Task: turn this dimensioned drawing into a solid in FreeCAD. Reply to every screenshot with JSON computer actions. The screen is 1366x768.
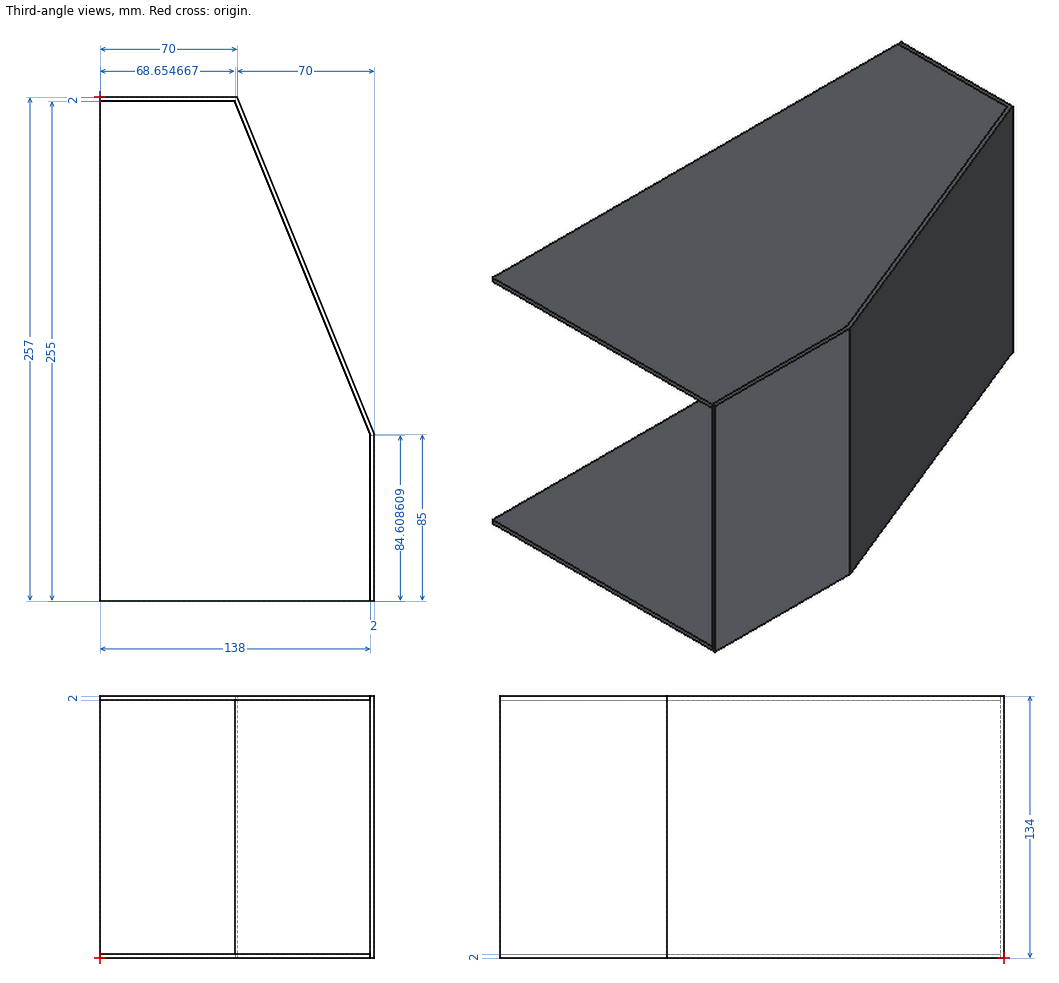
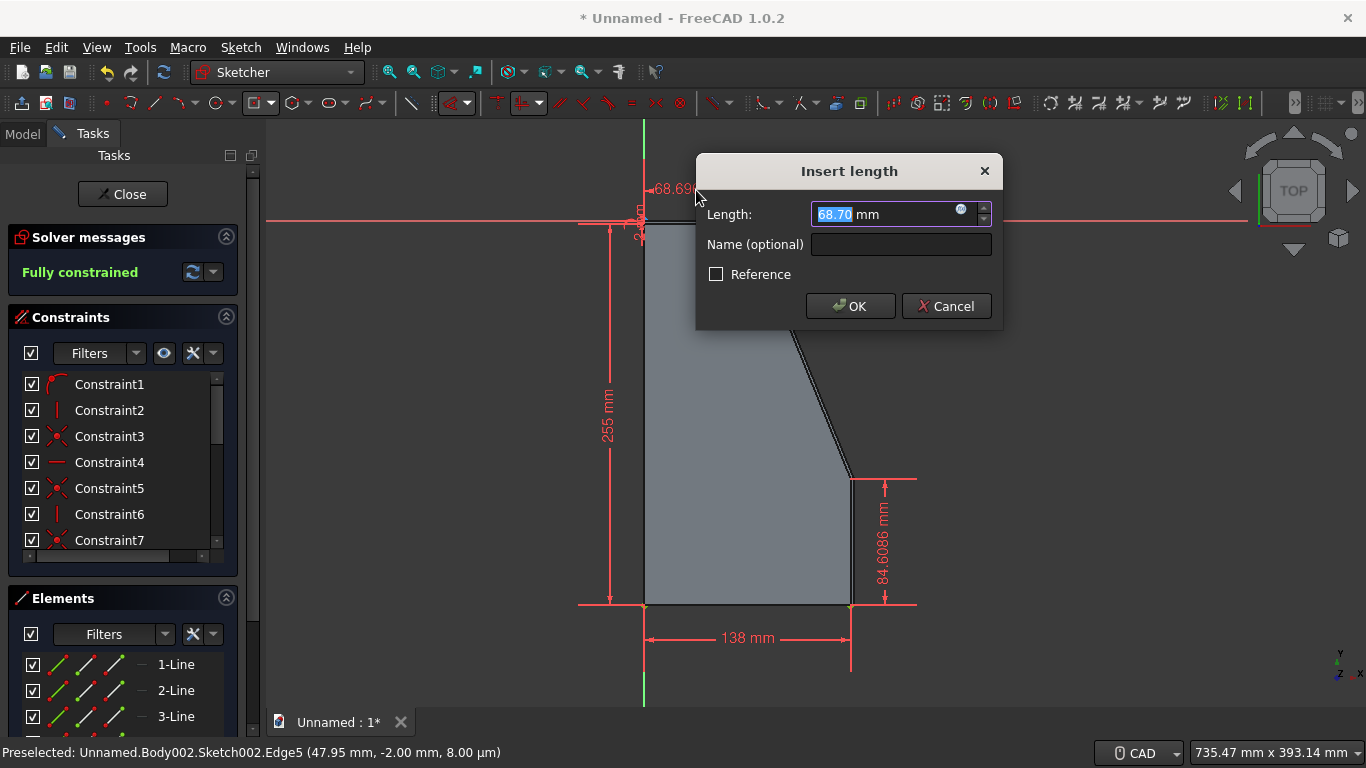
{"action": "type", "text": "68.654667"}
{"action": "key", "text": "Return"}
{"action": "key", "text": "Escape"}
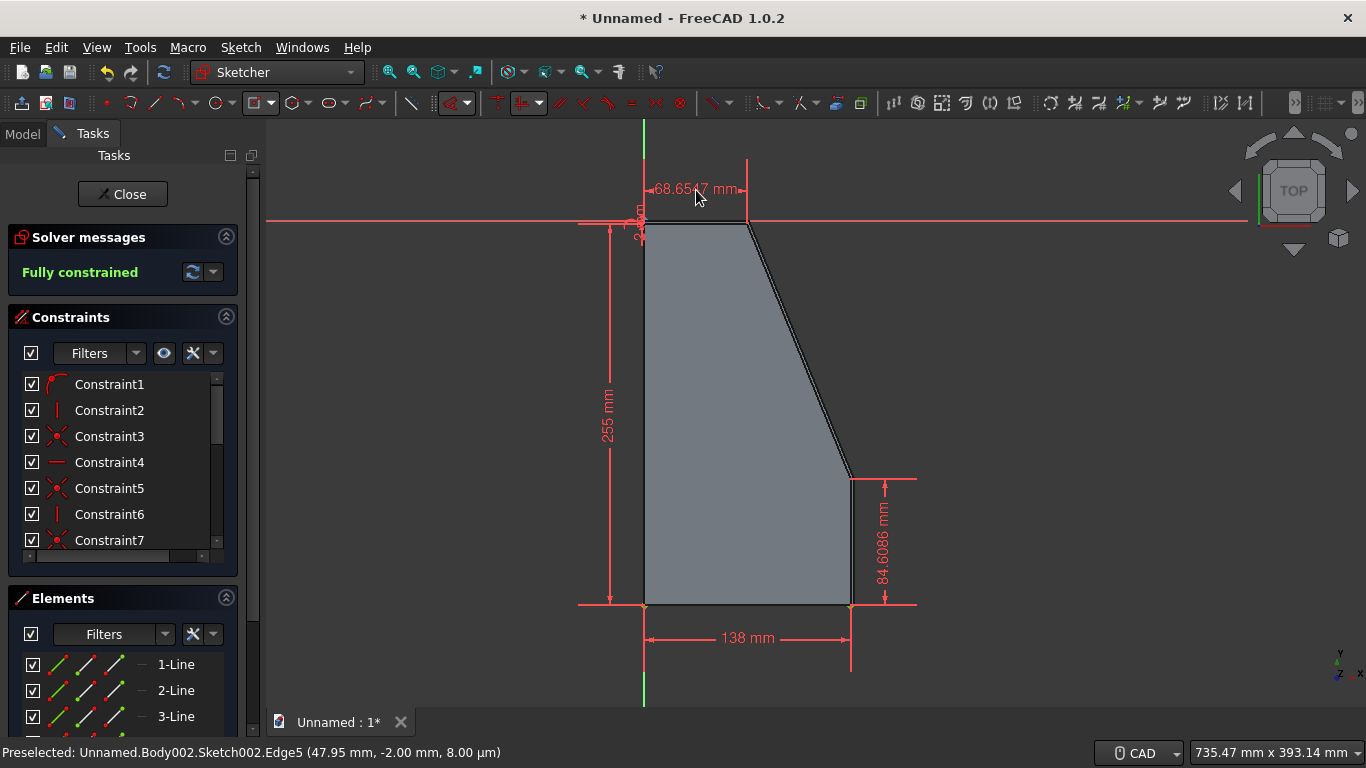
{"action": "left_click", "coordinate": [123, 194]}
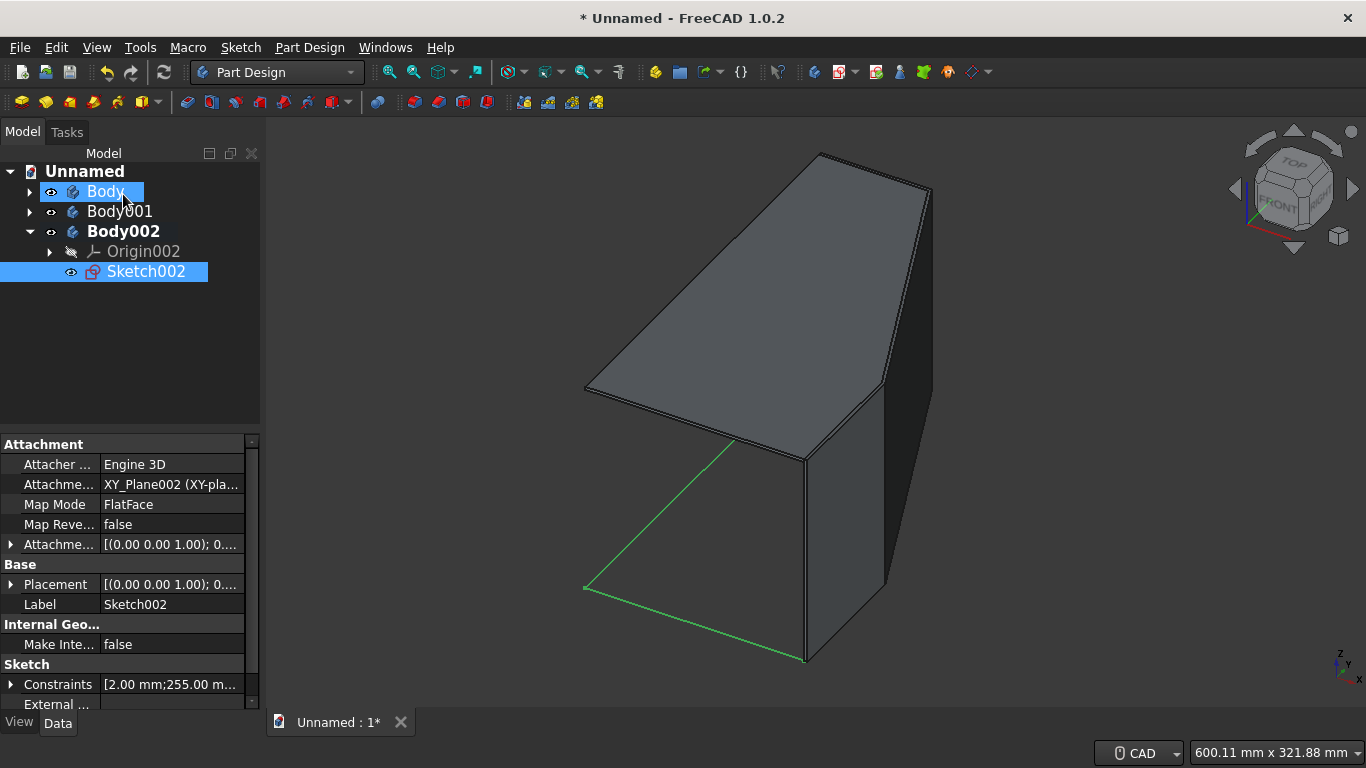
{"action": "left_click", "coordinate": [22, 102]}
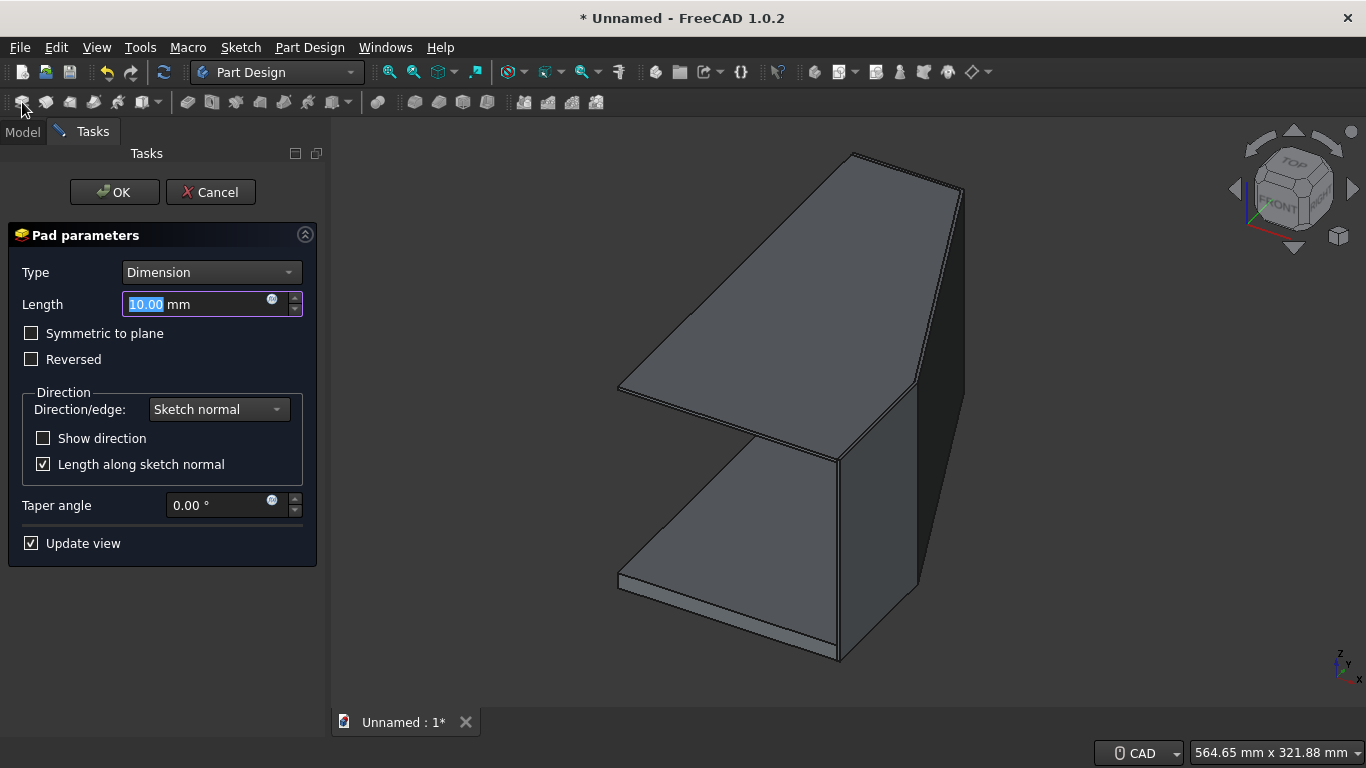
{"action": "type", "text": "2"}
{"action": "key", "text": "Tab"}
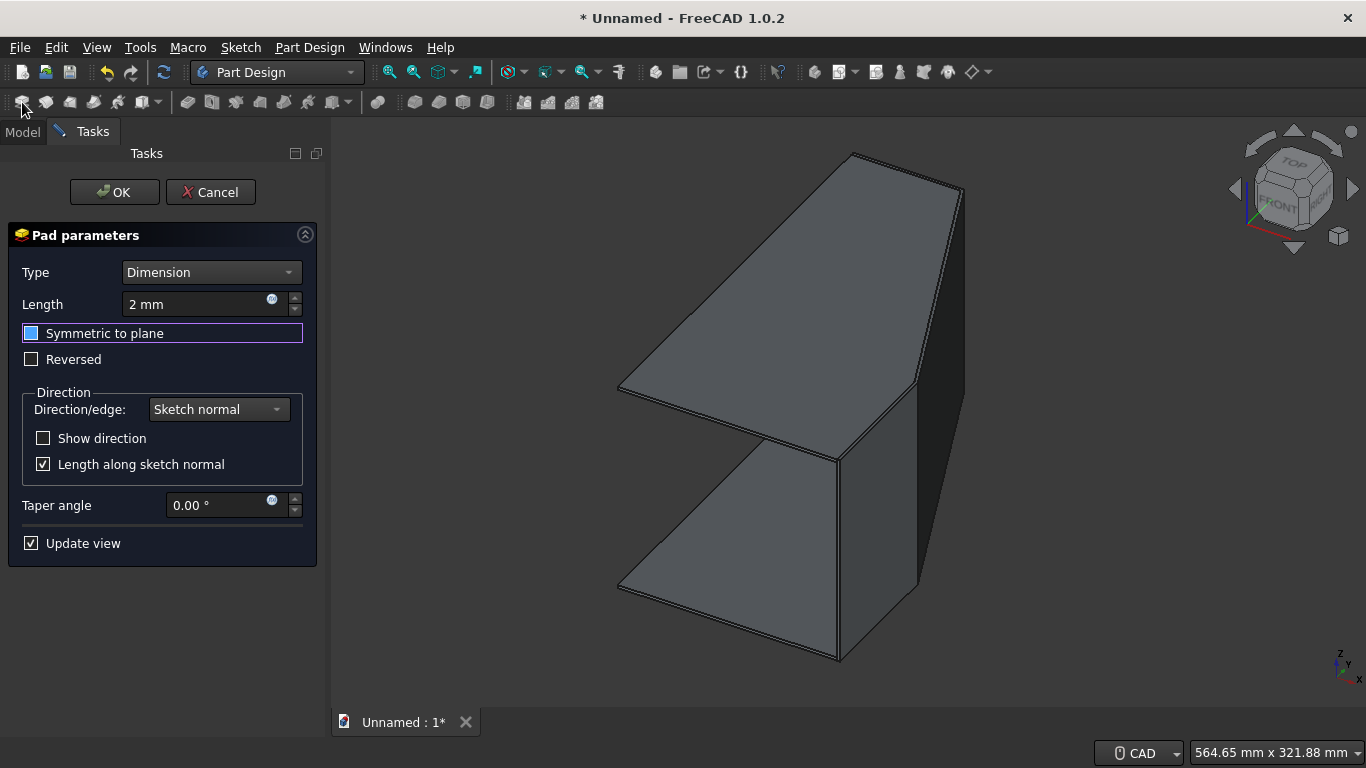
{"action": "left_click", "coordinate": [115, 192]}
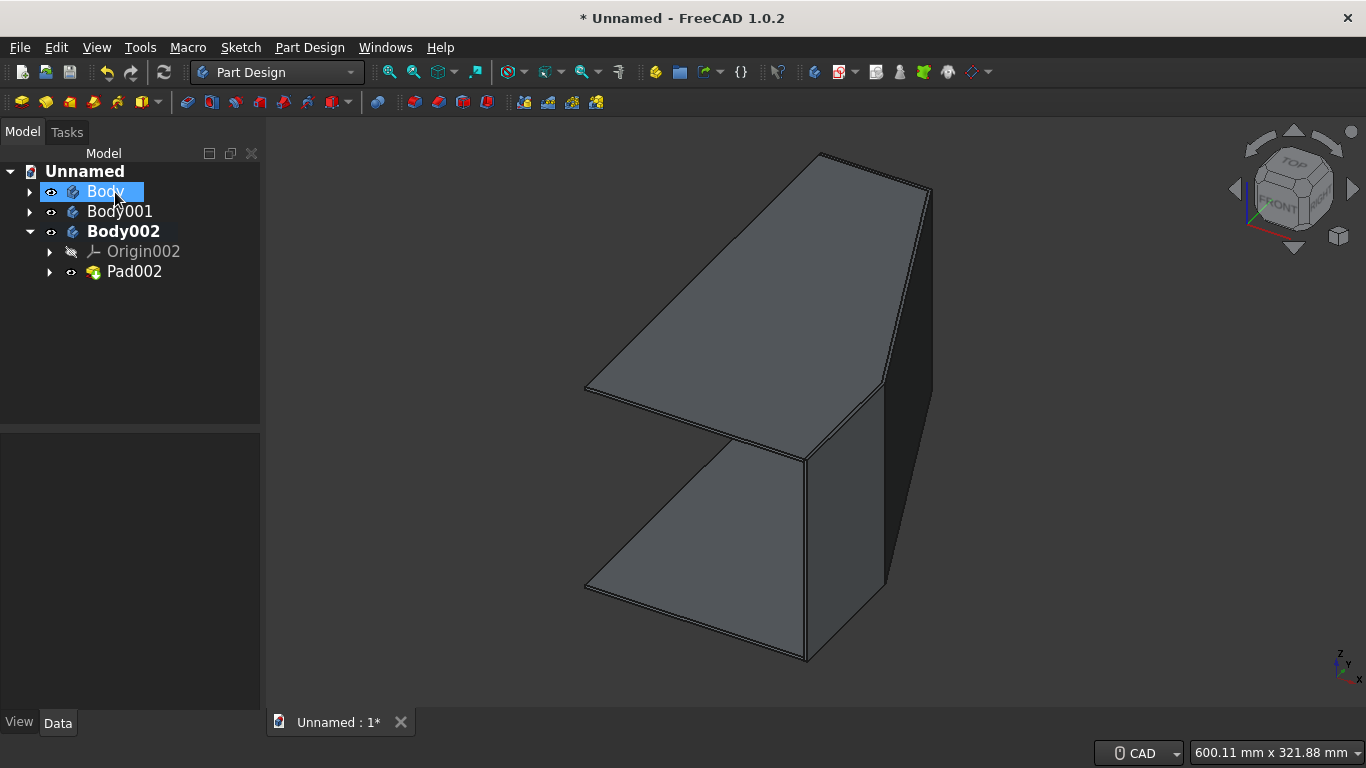
{"action": "key", "text": "0"}